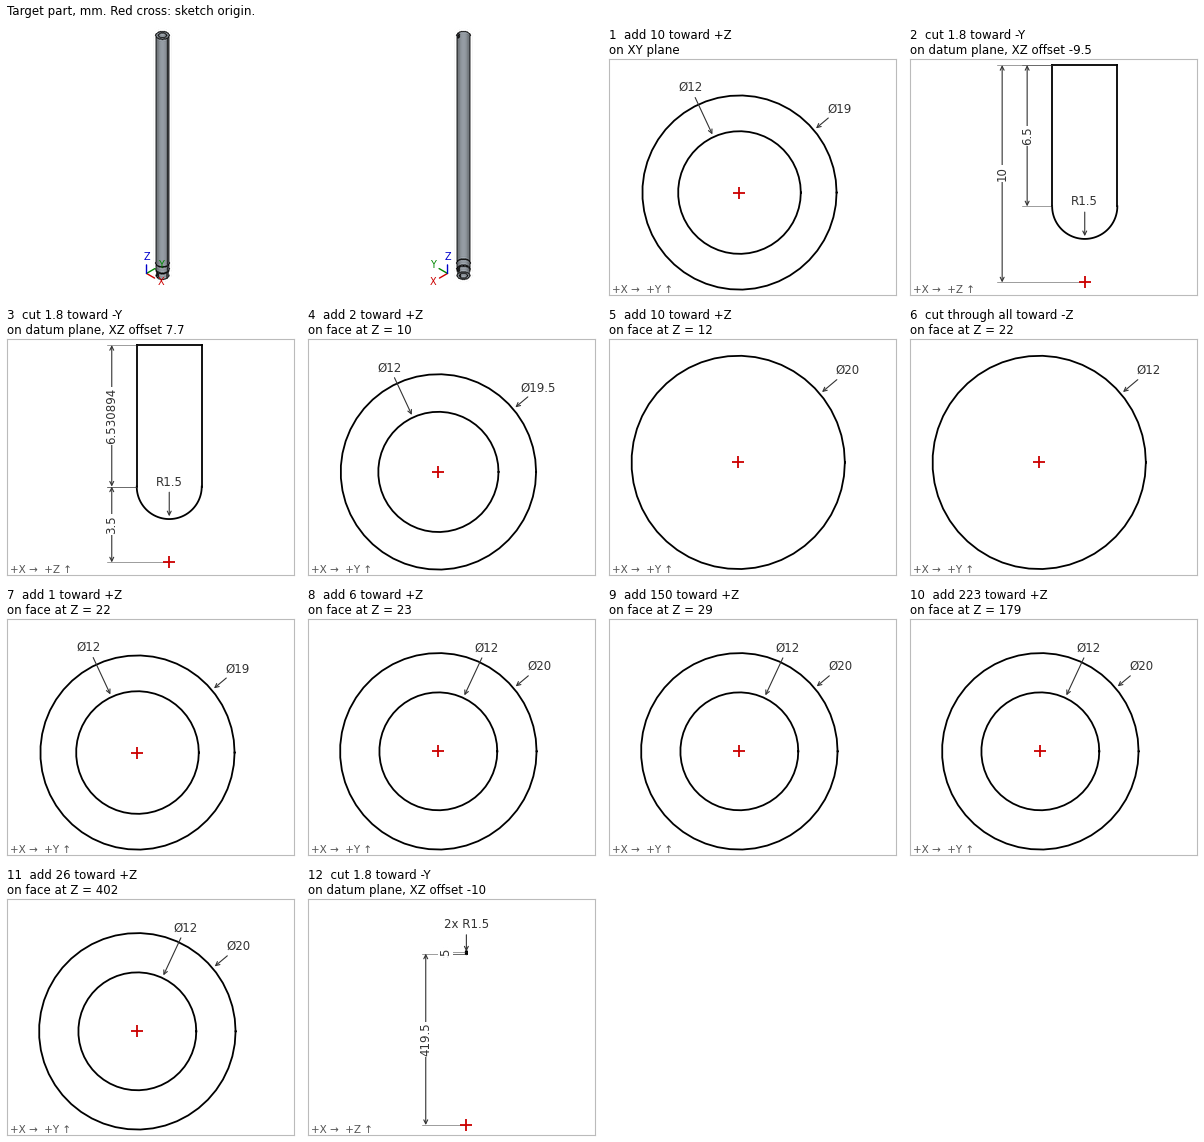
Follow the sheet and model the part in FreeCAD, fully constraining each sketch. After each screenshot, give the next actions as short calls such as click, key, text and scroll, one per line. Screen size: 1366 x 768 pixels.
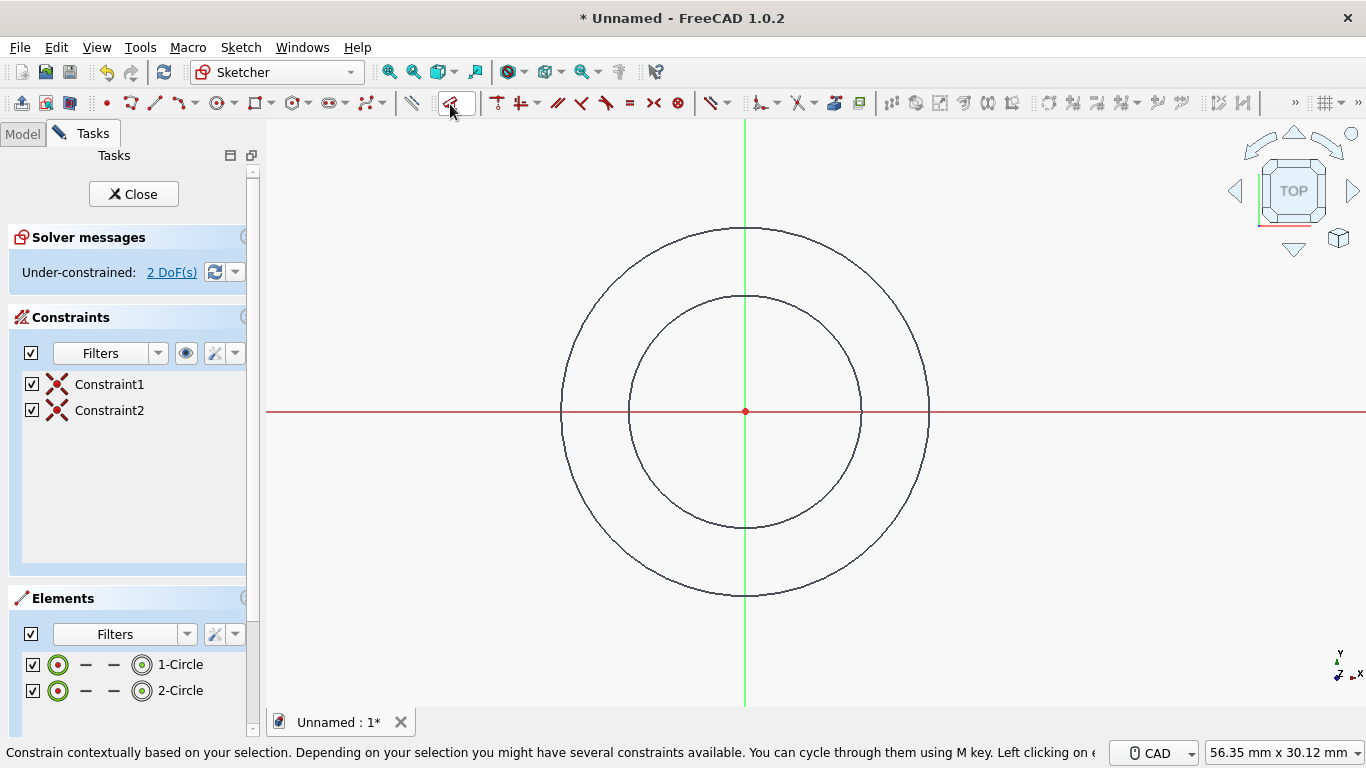
click(875, 281)
click(898, 258)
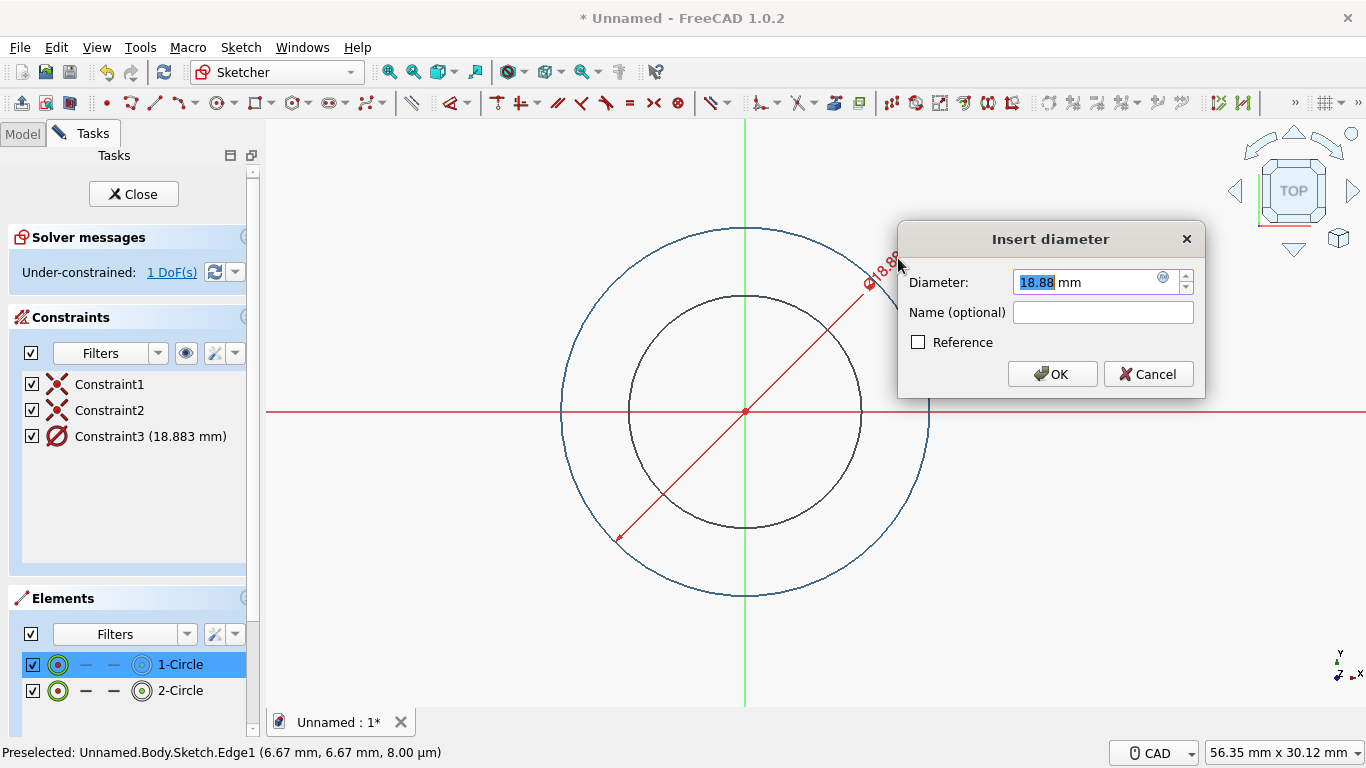
text(19)
key(Return)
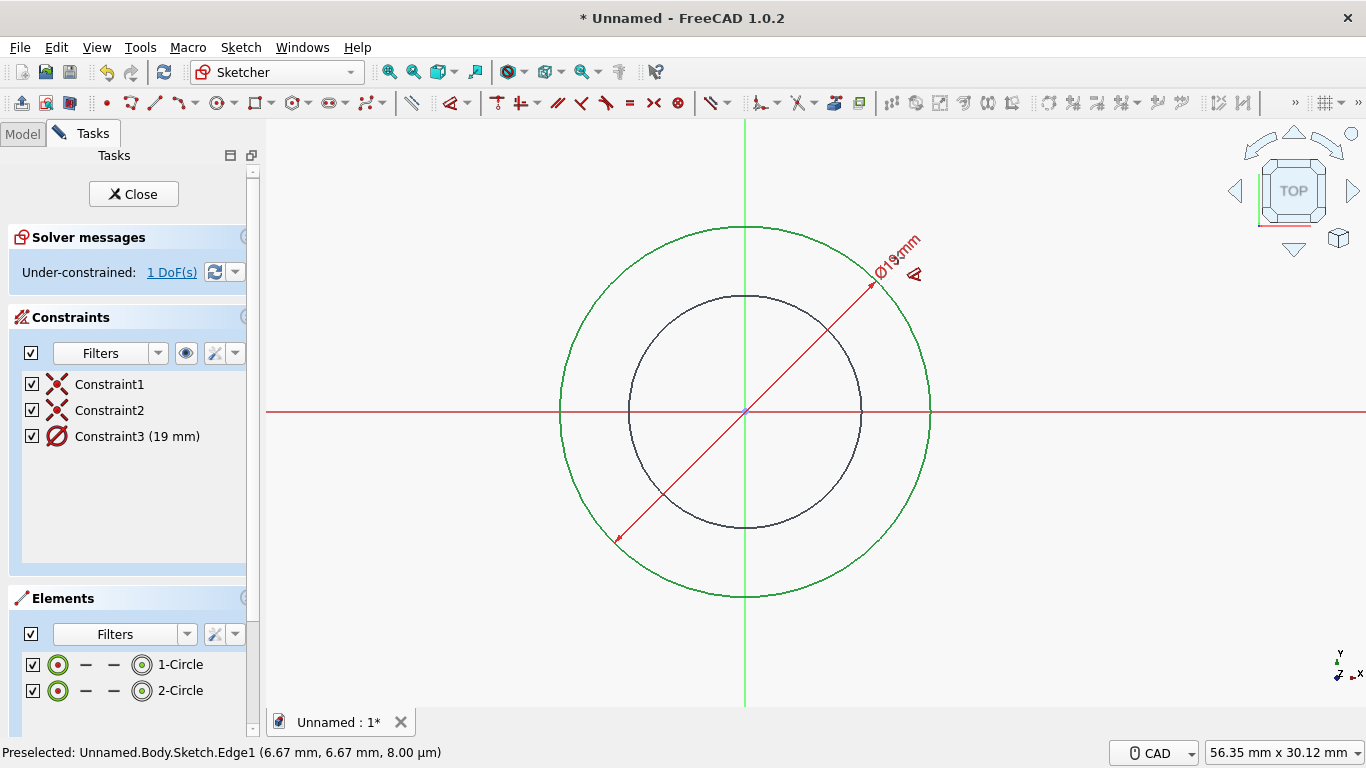
click(827, 329)
click(849, 306)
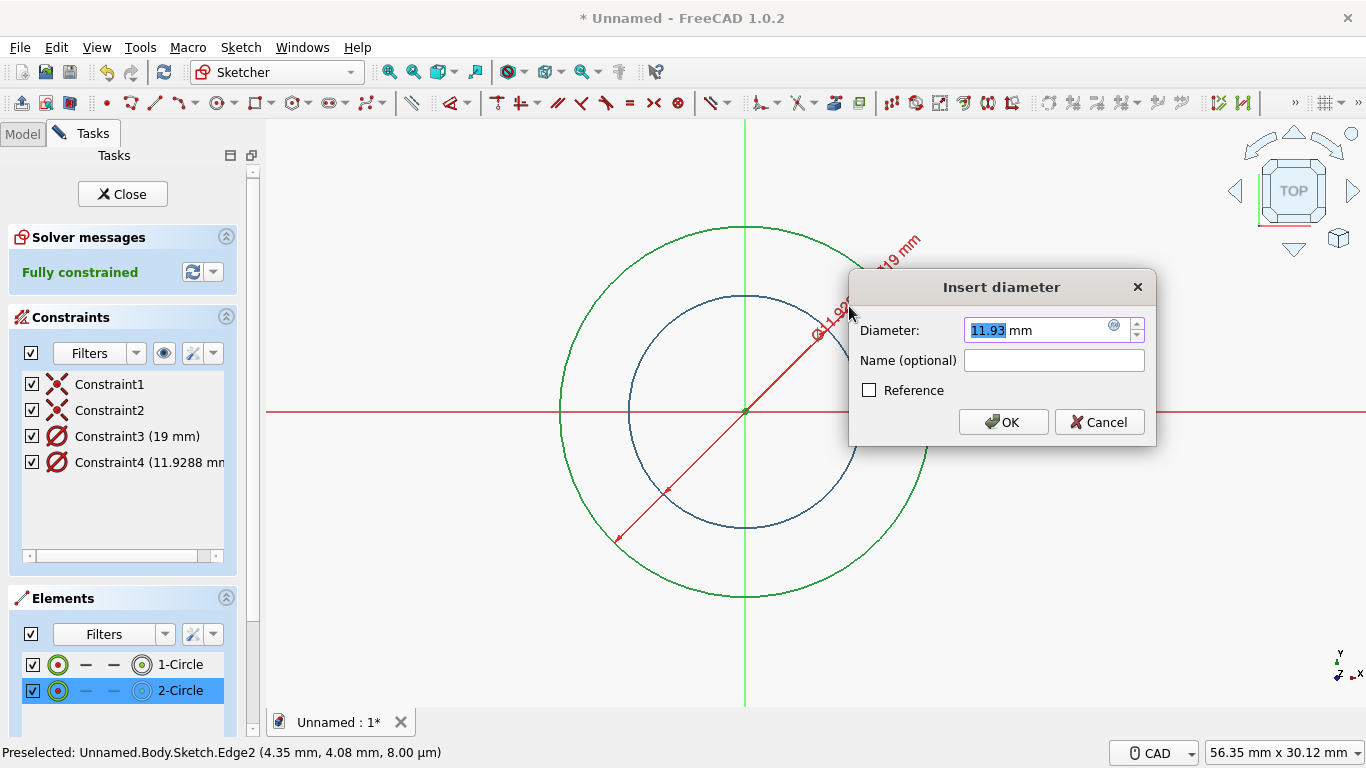
text(12)
key(Return)
key(Escape)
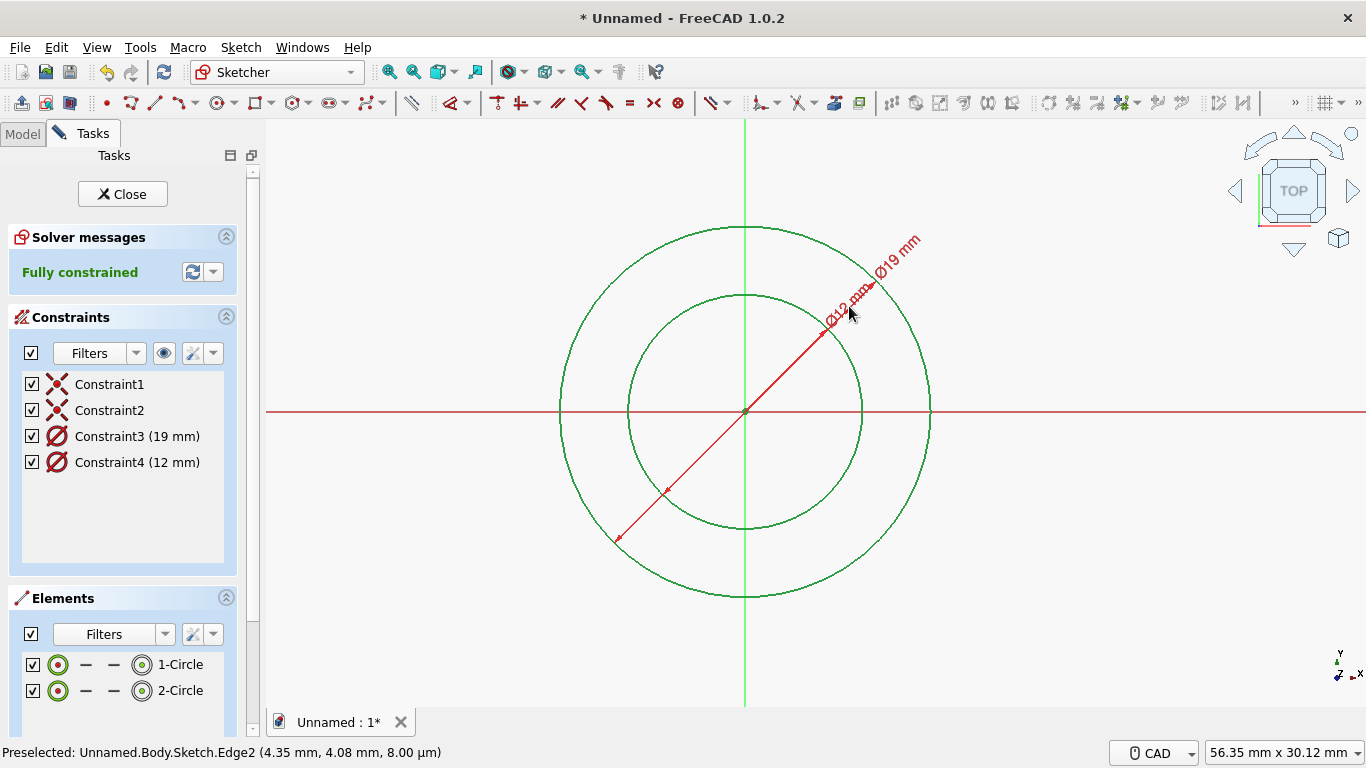
click(123, 194)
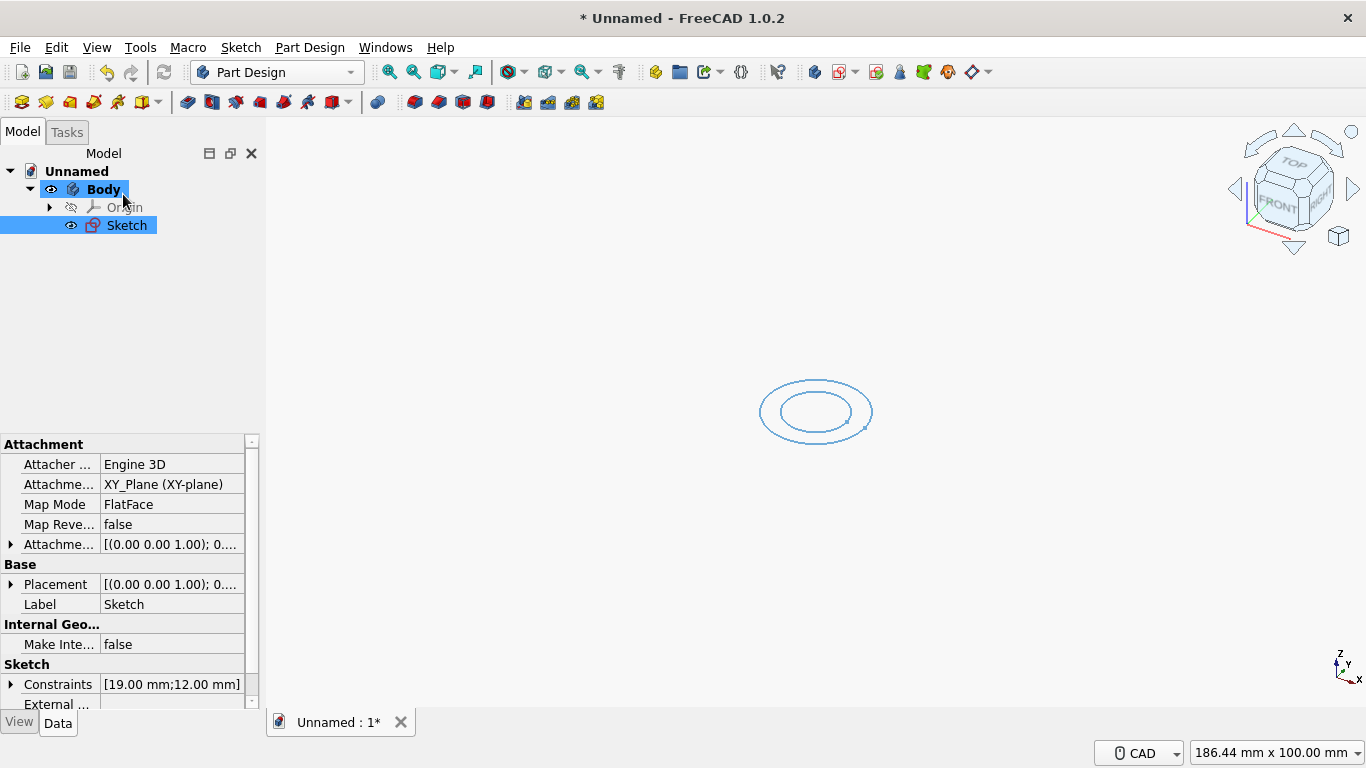
click(22, 102)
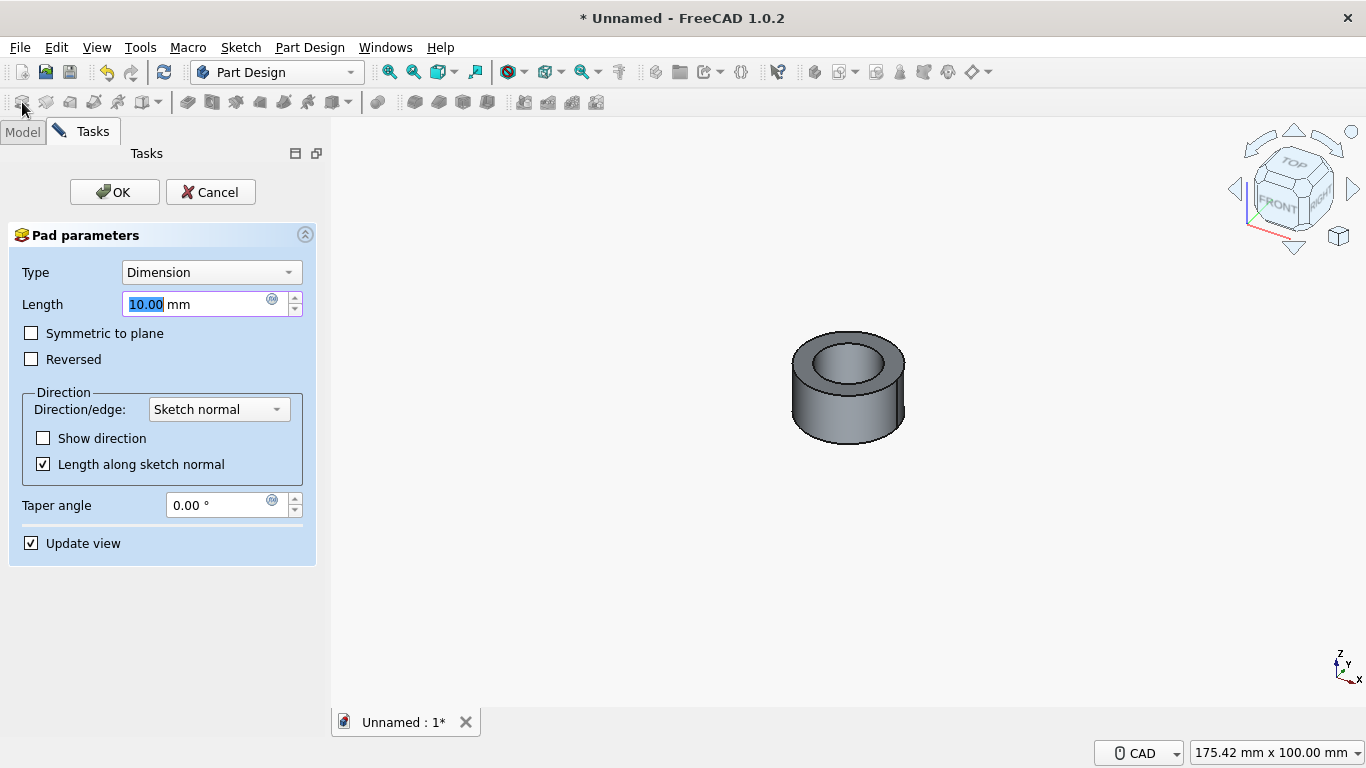
text(10)
key(Tab)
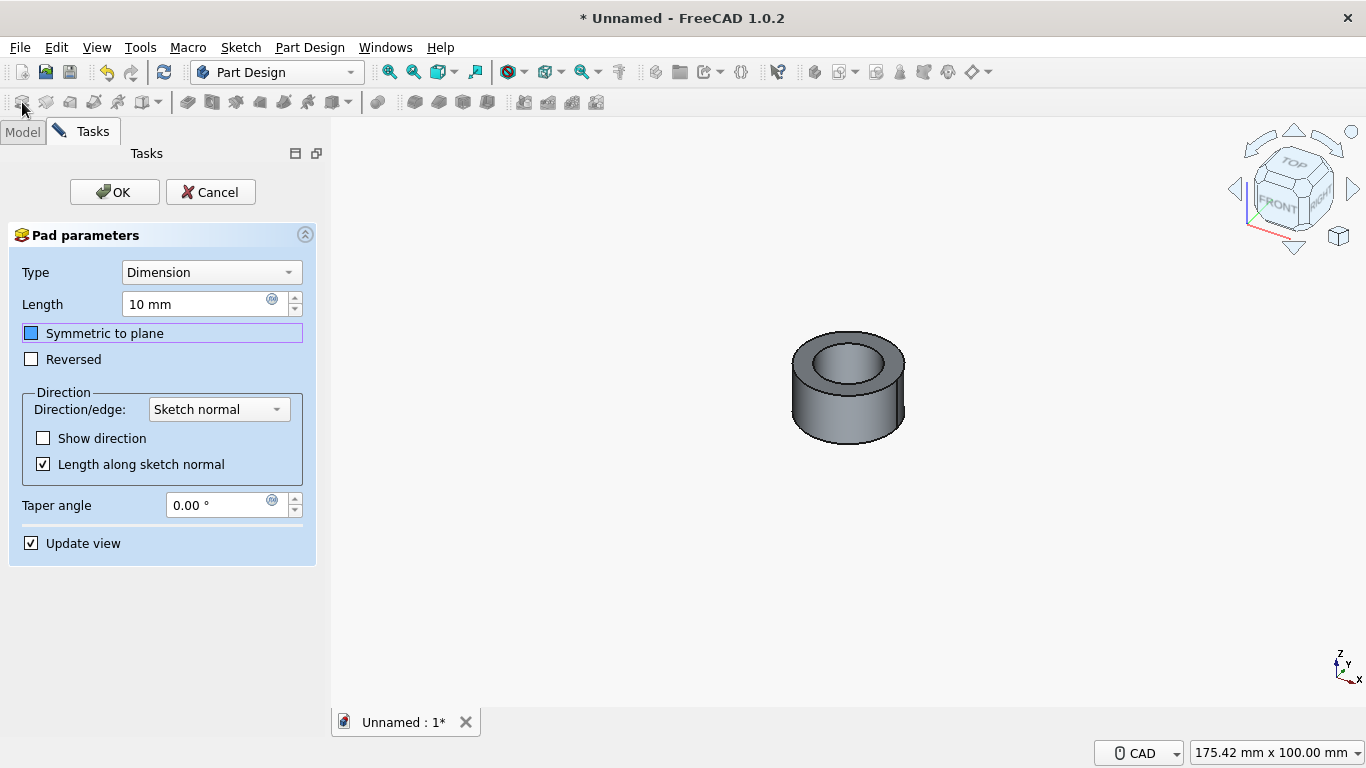
click(115, 192)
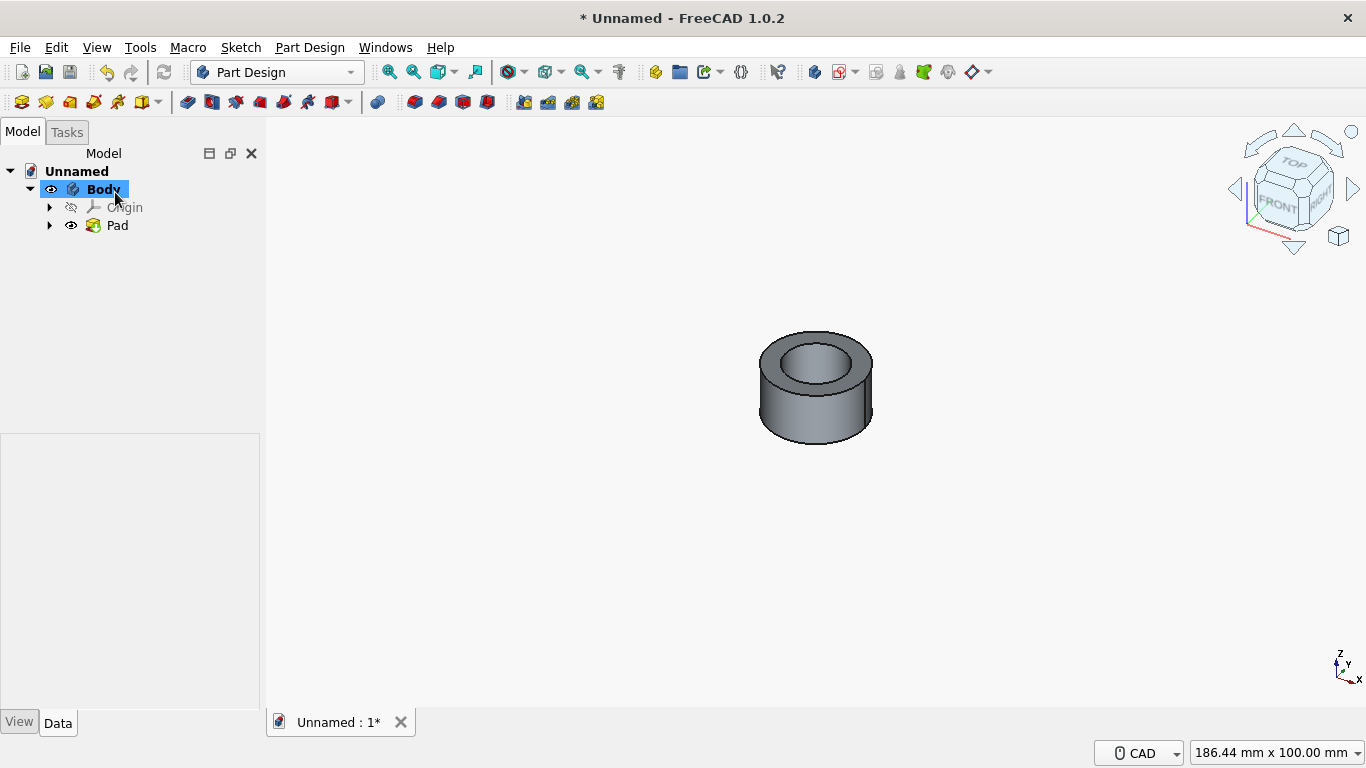
click(390, 72)